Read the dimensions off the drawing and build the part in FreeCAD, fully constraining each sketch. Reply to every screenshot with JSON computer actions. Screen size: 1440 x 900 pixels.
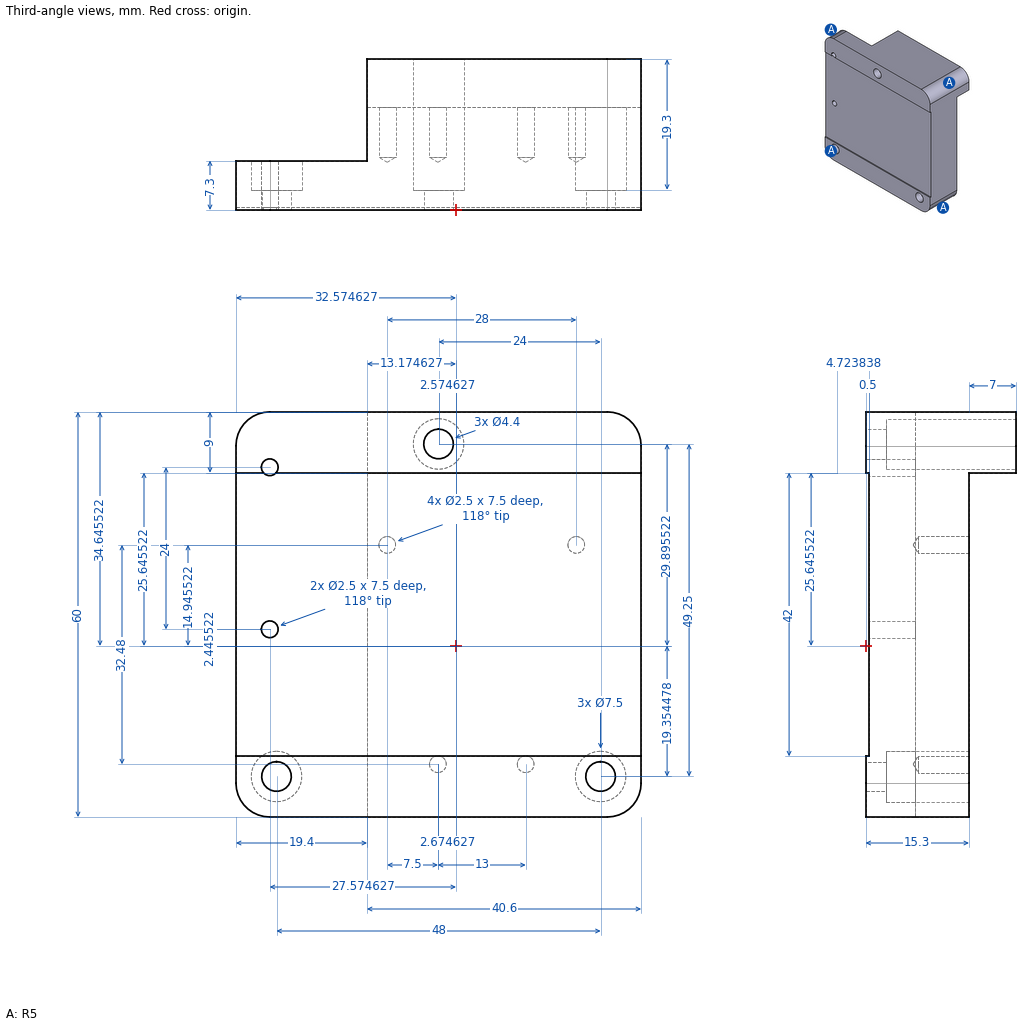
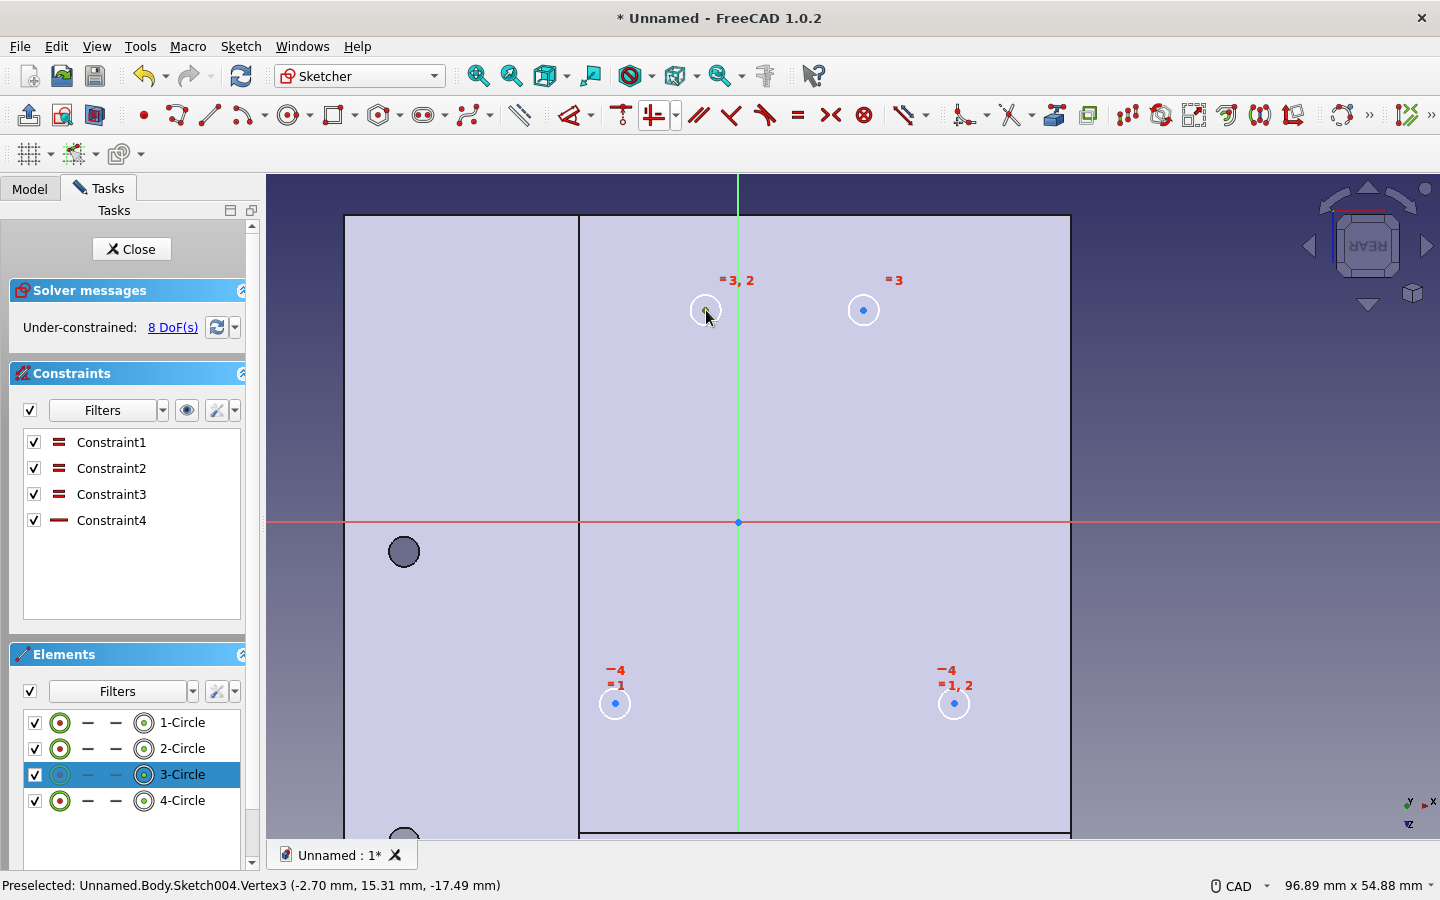
{"action": "left_click", "coordinate": [864, 310]}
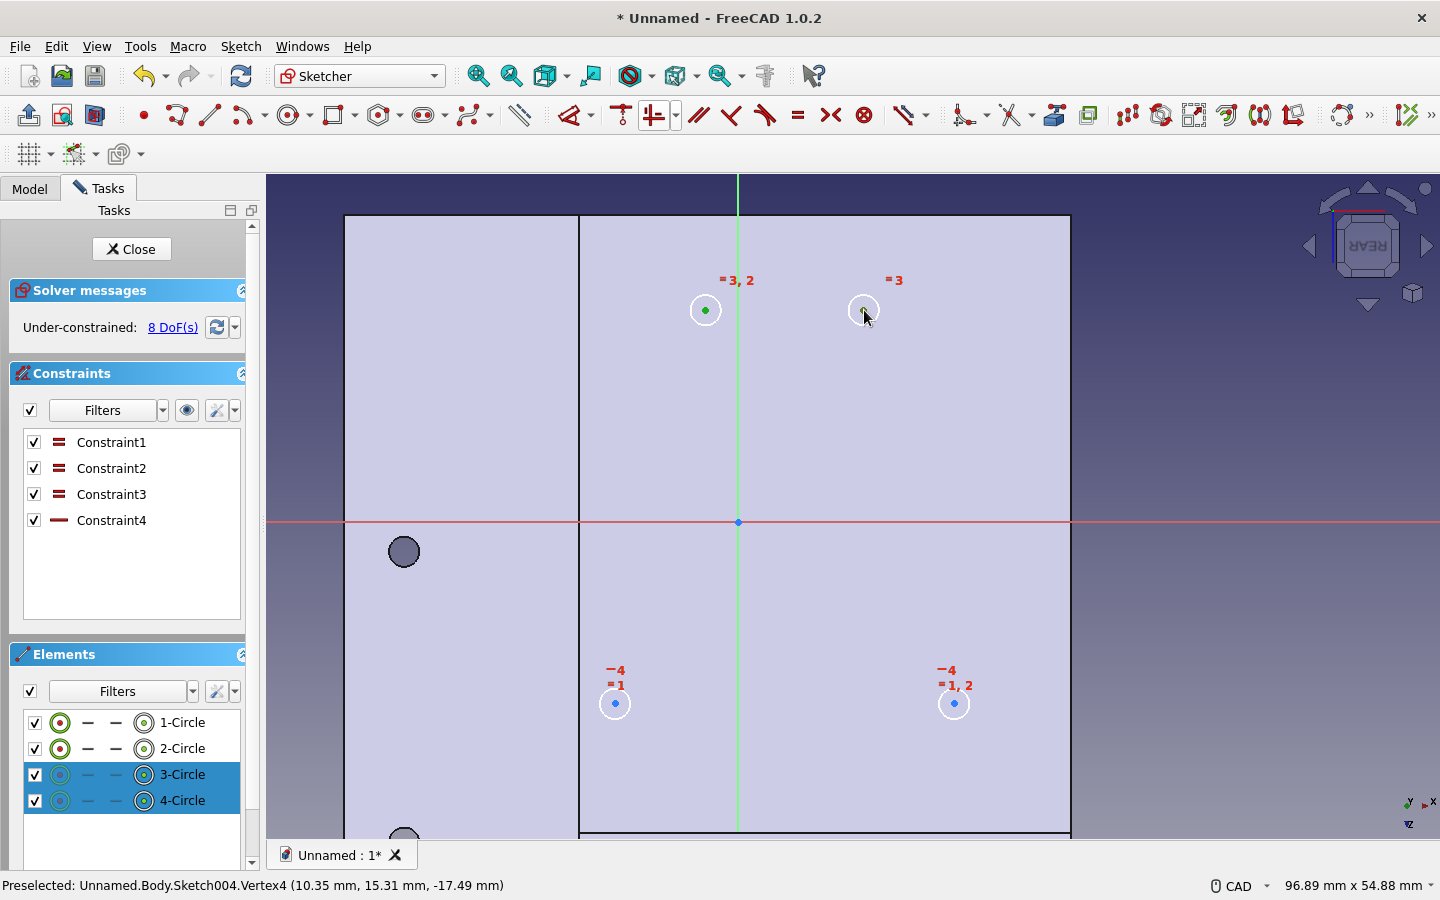
{"action": "key", "text": "h"}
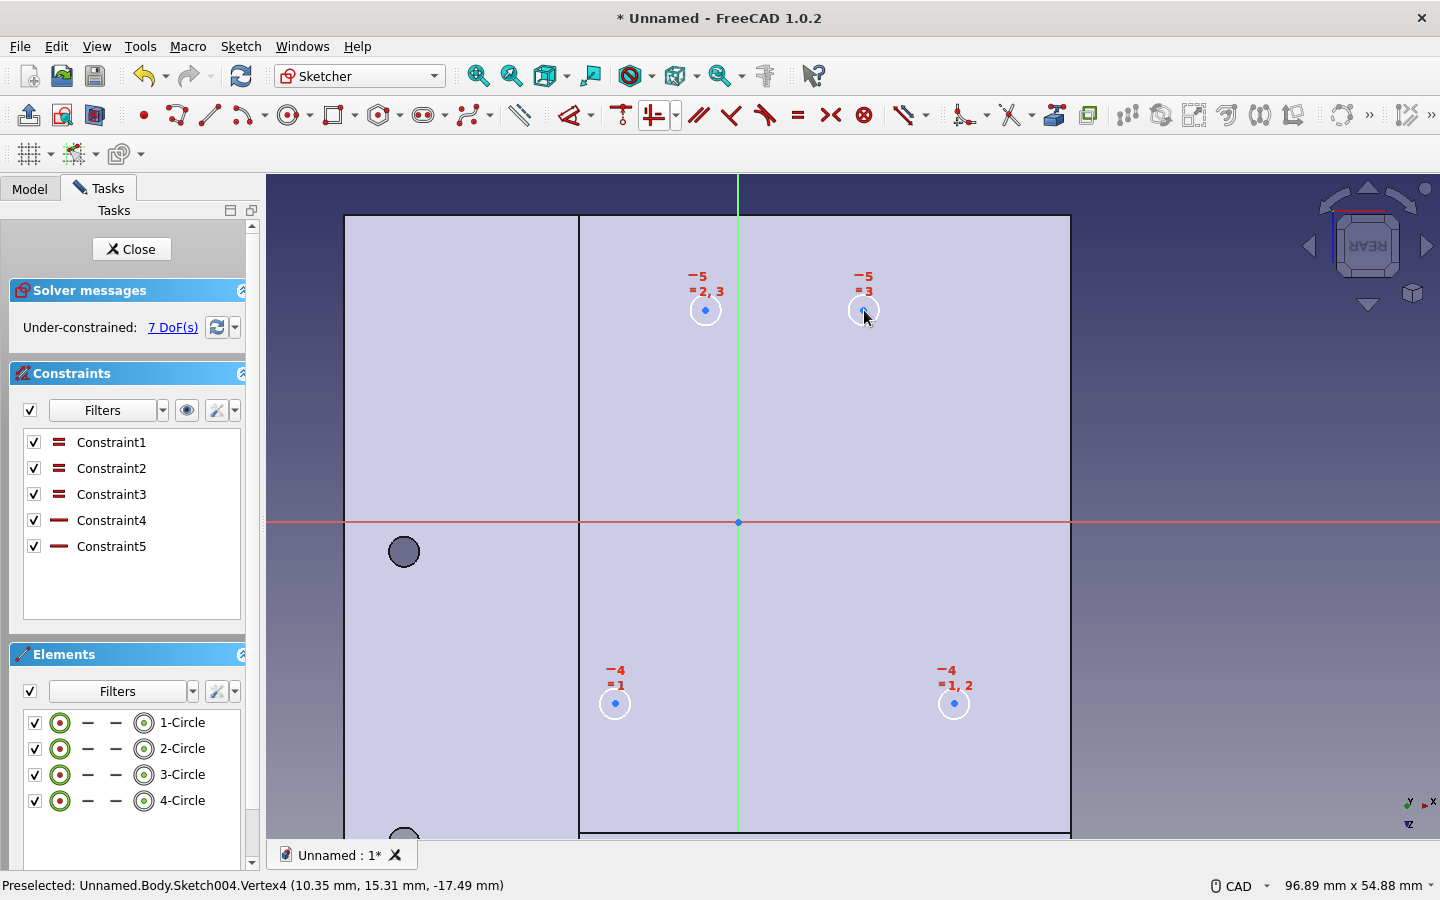
{"action": "left_click", "coordinate": [568, 116]}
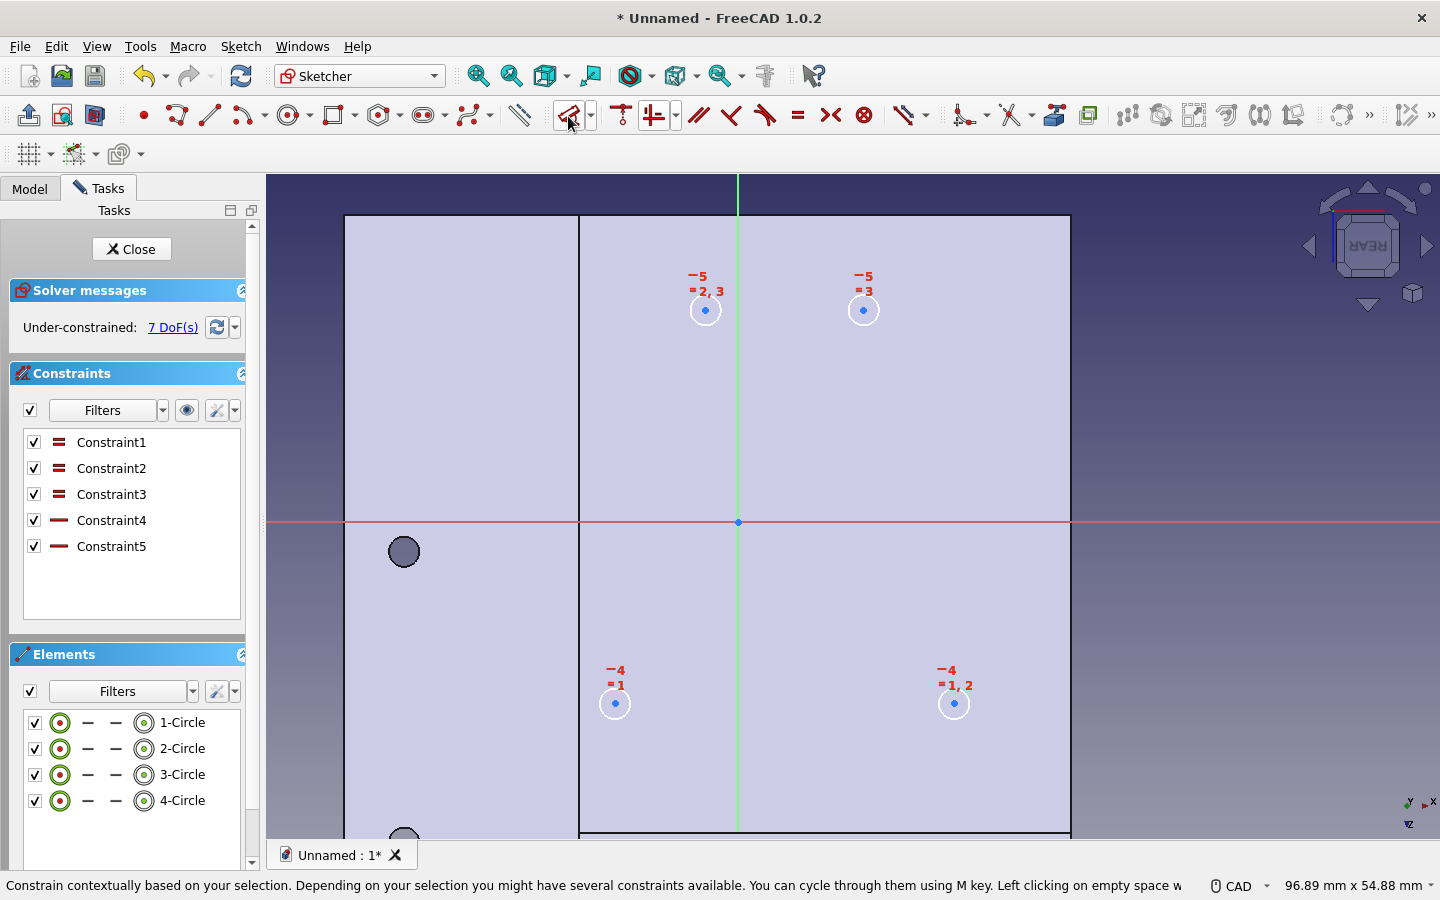
{"action": "scroll", "coordinate": [626, 693], "scroll_direction": "up", "scroll_amount": 2}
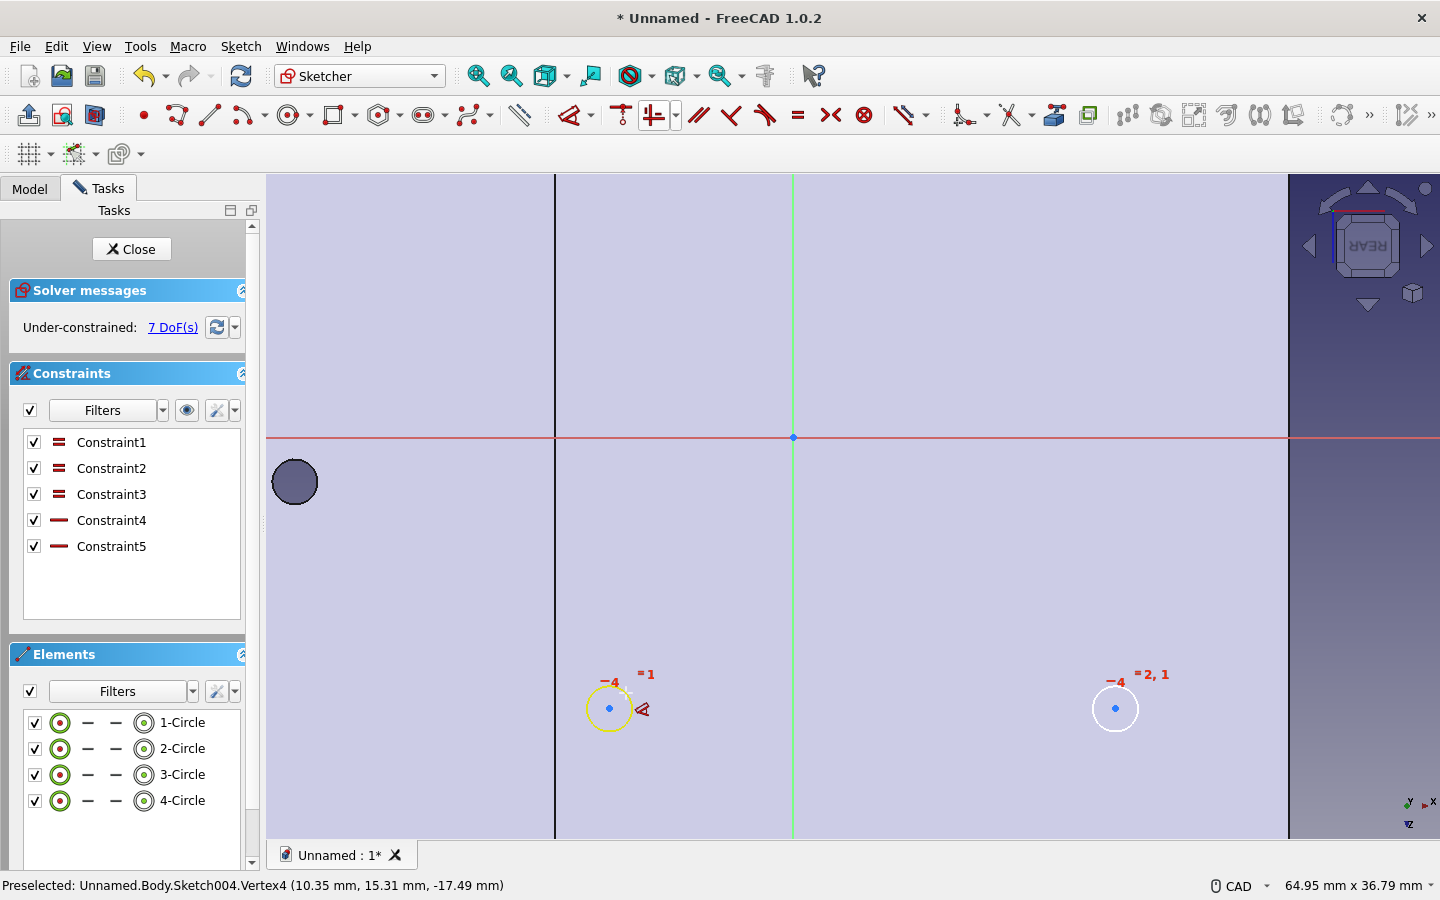
{"action": "left_click", "coordinate": [625, 693]}
{"action": "left_click", "coordinate": [647, 670]}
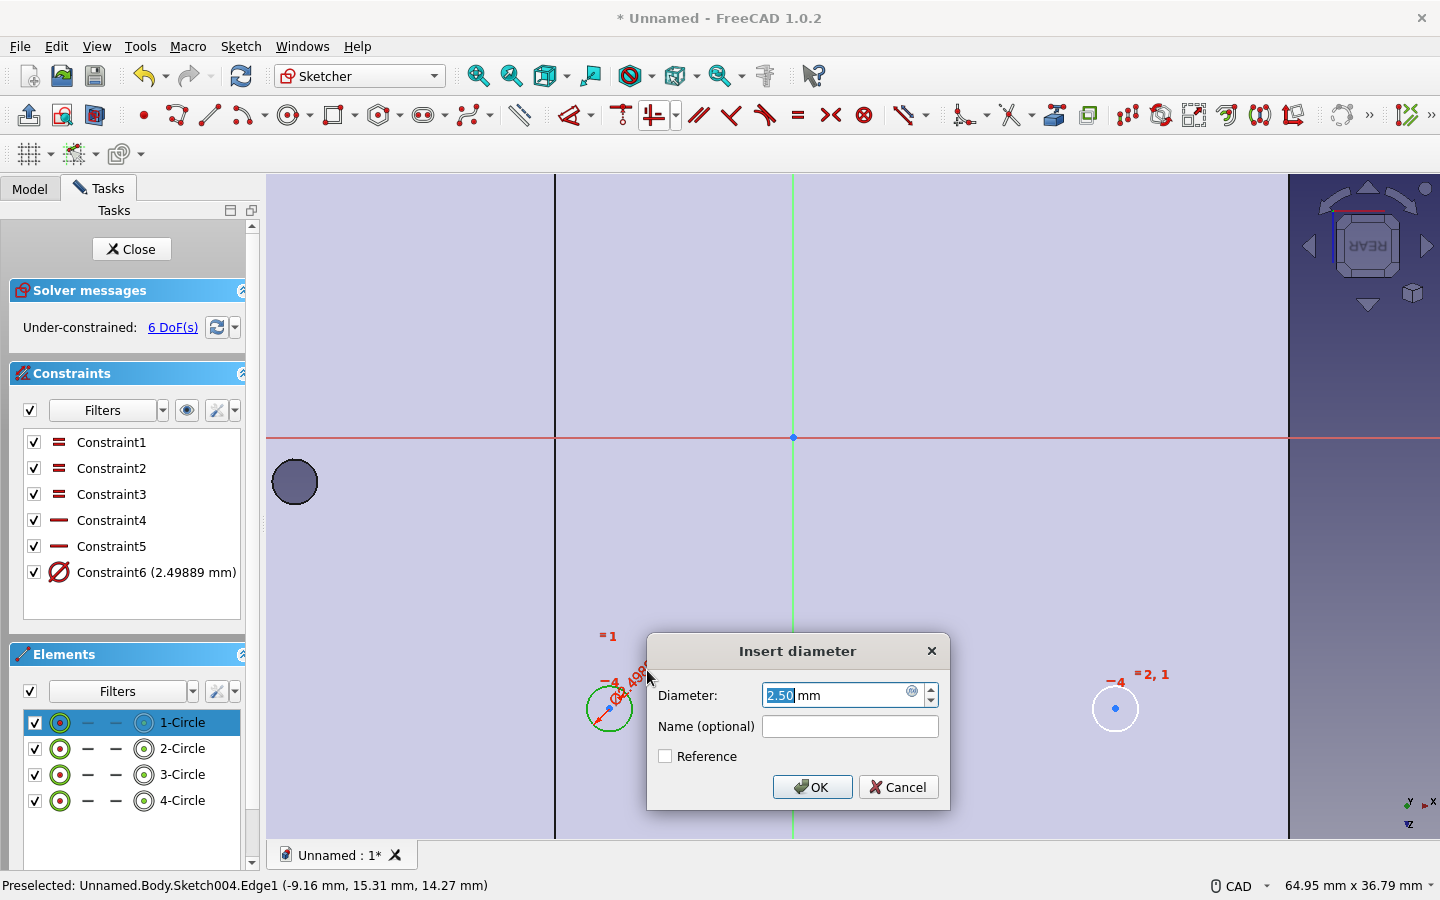
{"action": "type", "text": "2.5"}
{"action": "key", "text": "Return"}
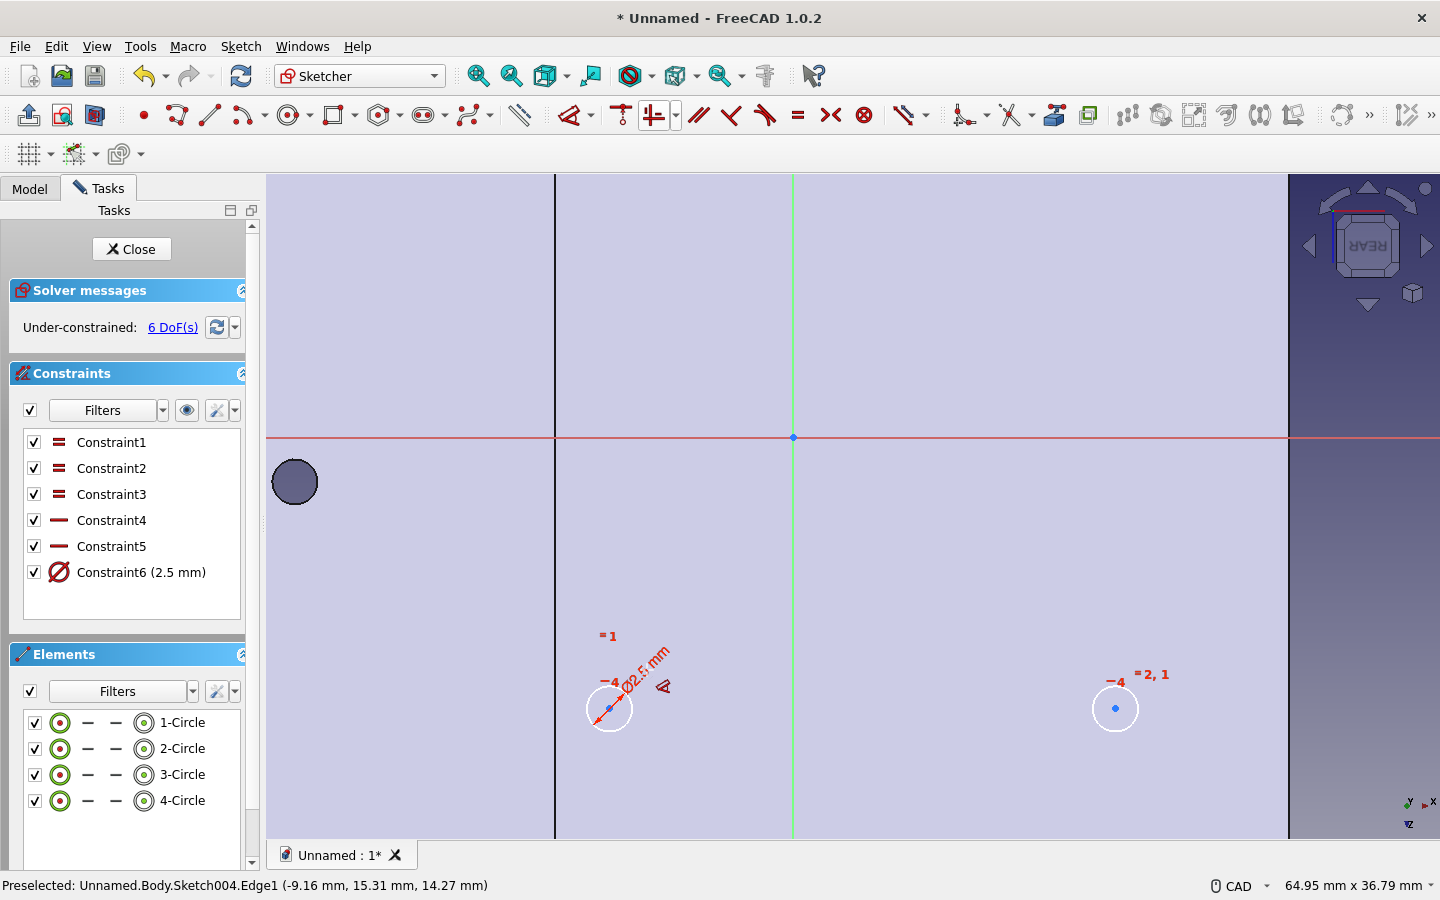
{"action": "left_click", "coordinate": [609, 709]}